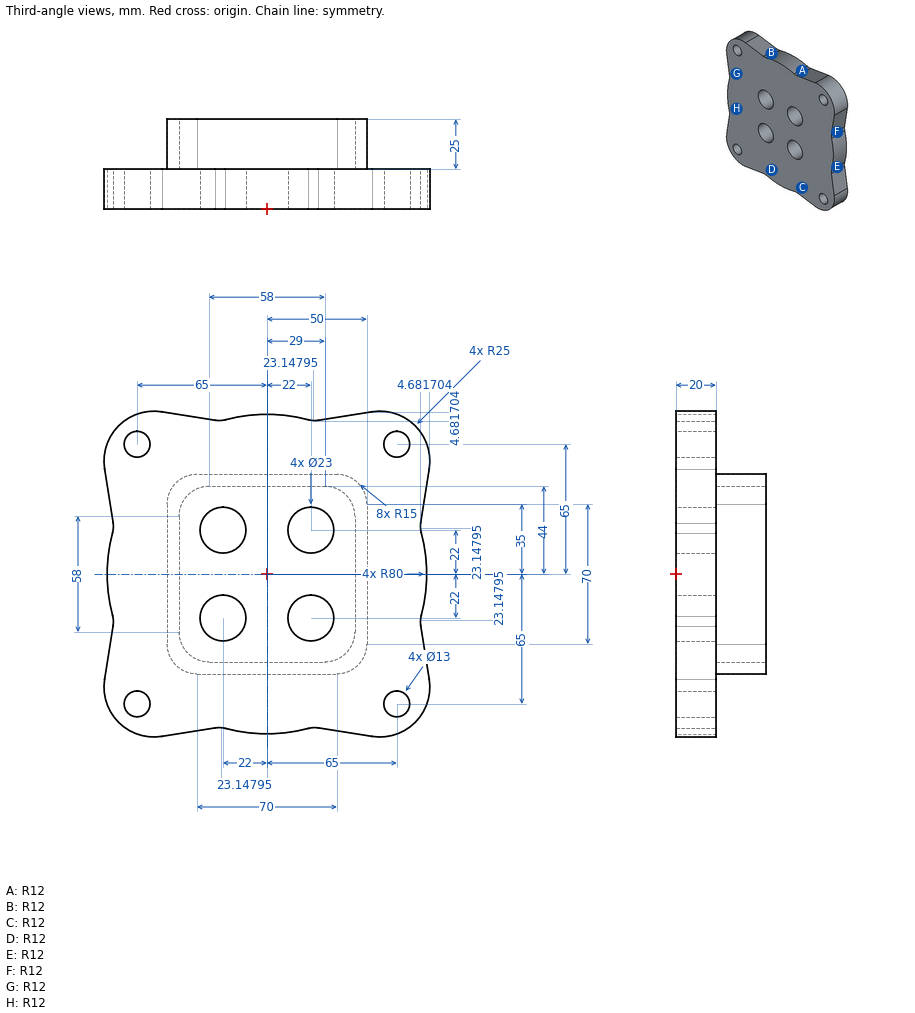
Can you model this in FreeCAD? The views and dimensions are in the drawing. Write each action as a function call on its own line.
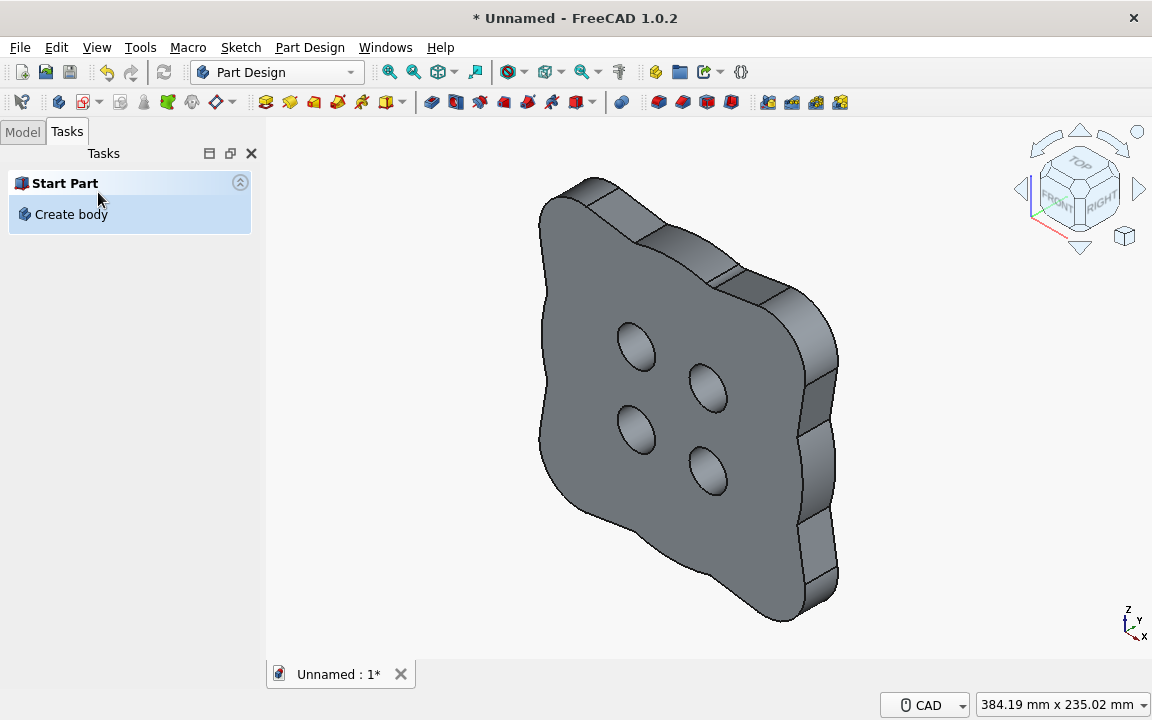
key(2)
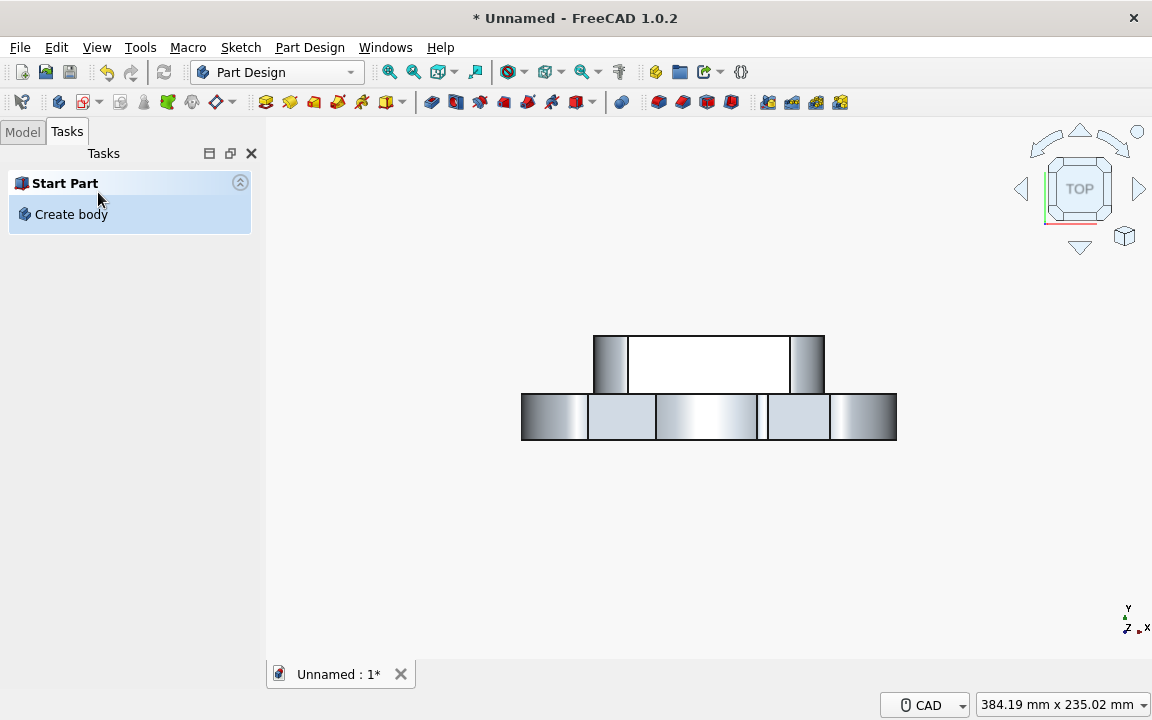
click(390, 72)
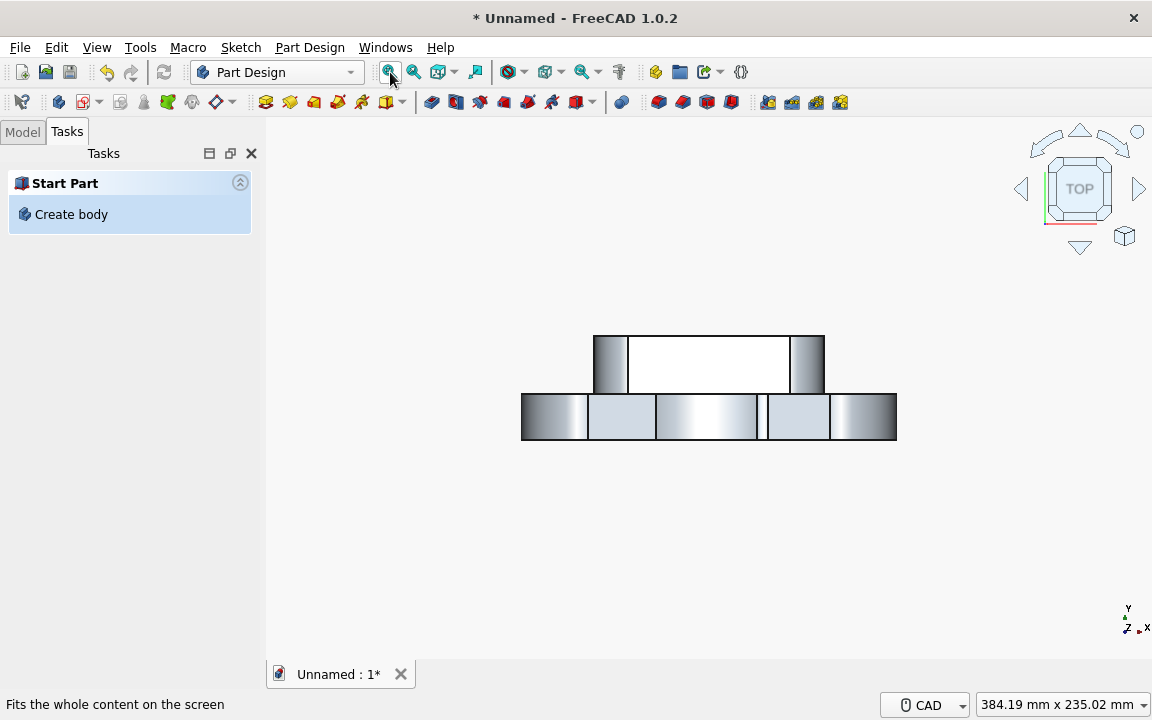
key(0)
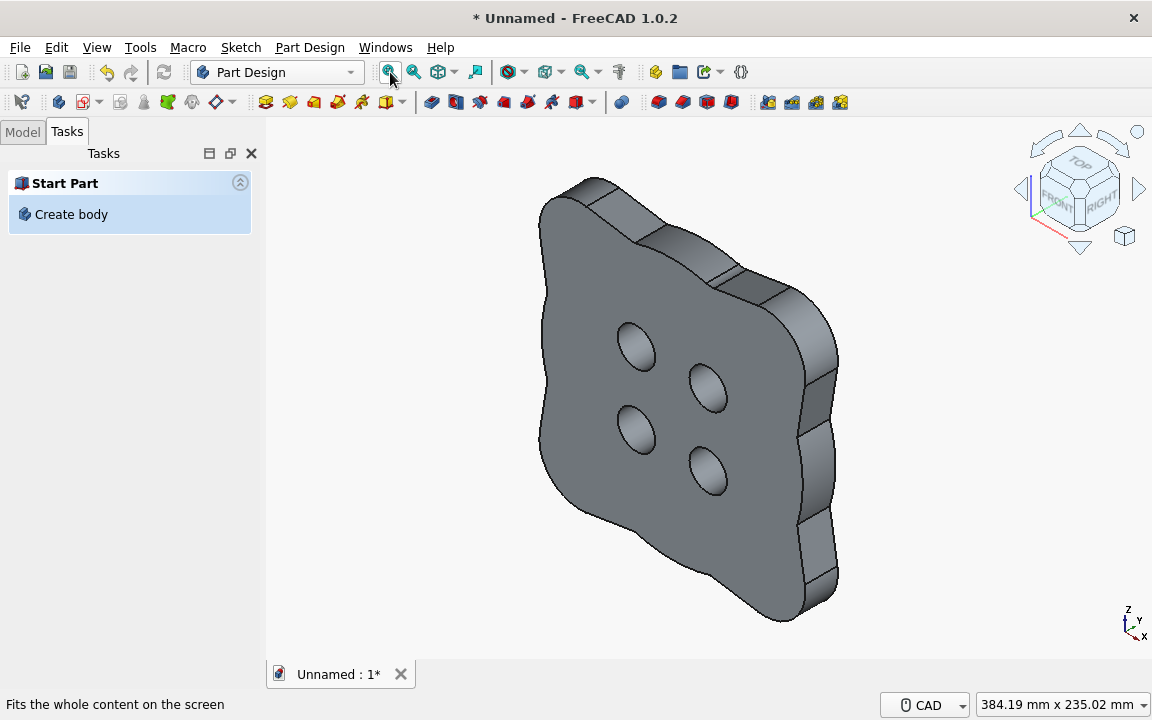
key(1)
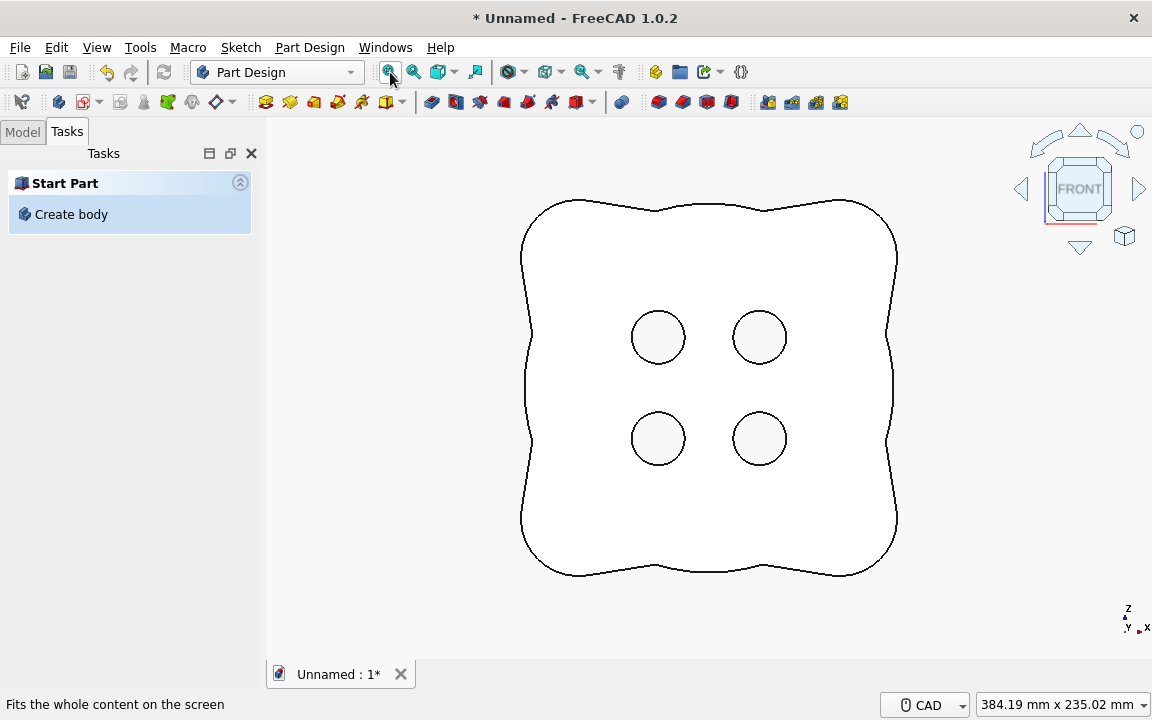
key(3)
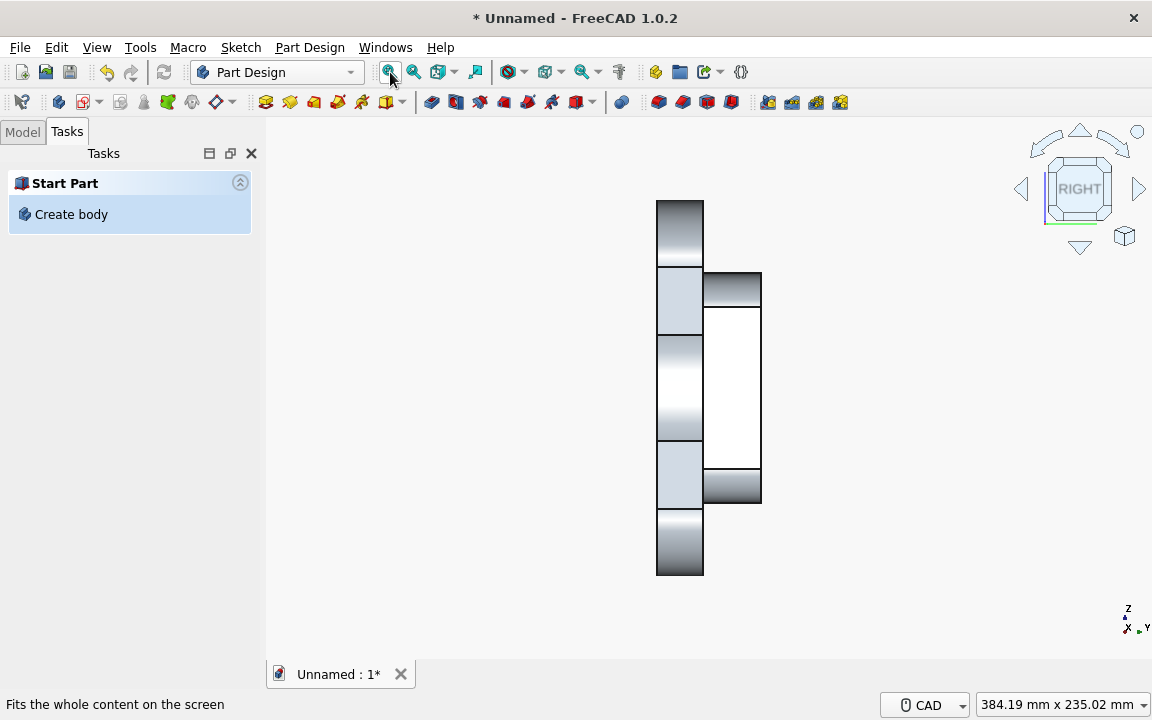
key(5)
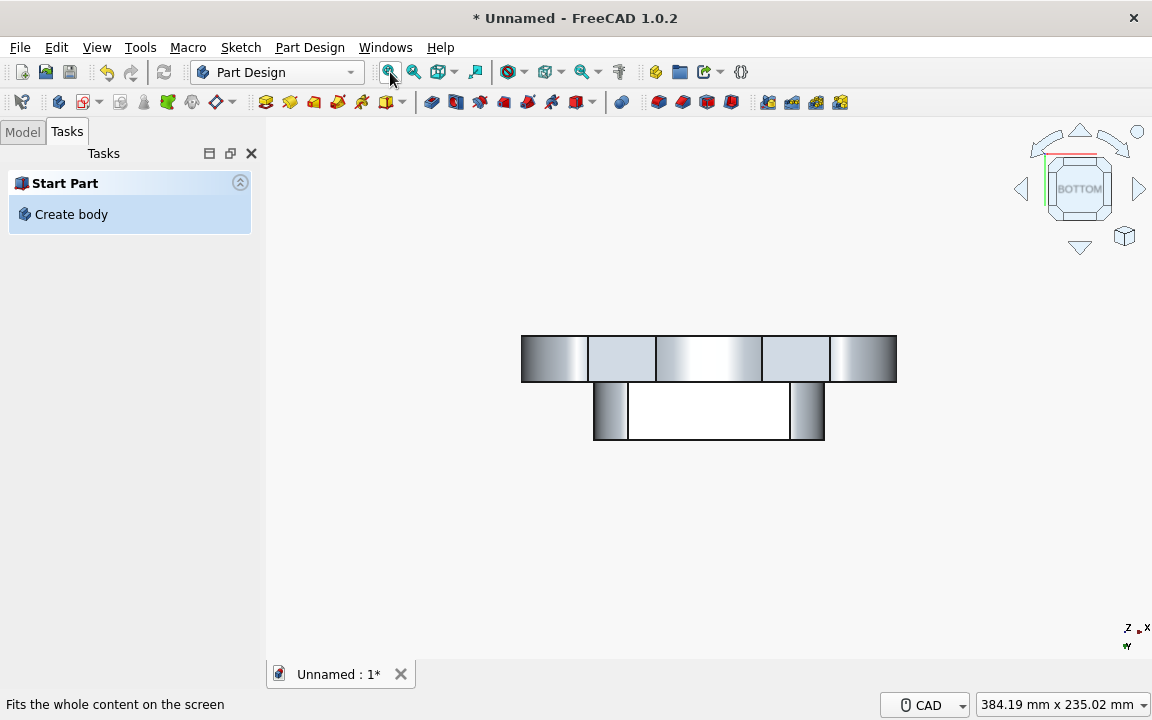
click(390, 72)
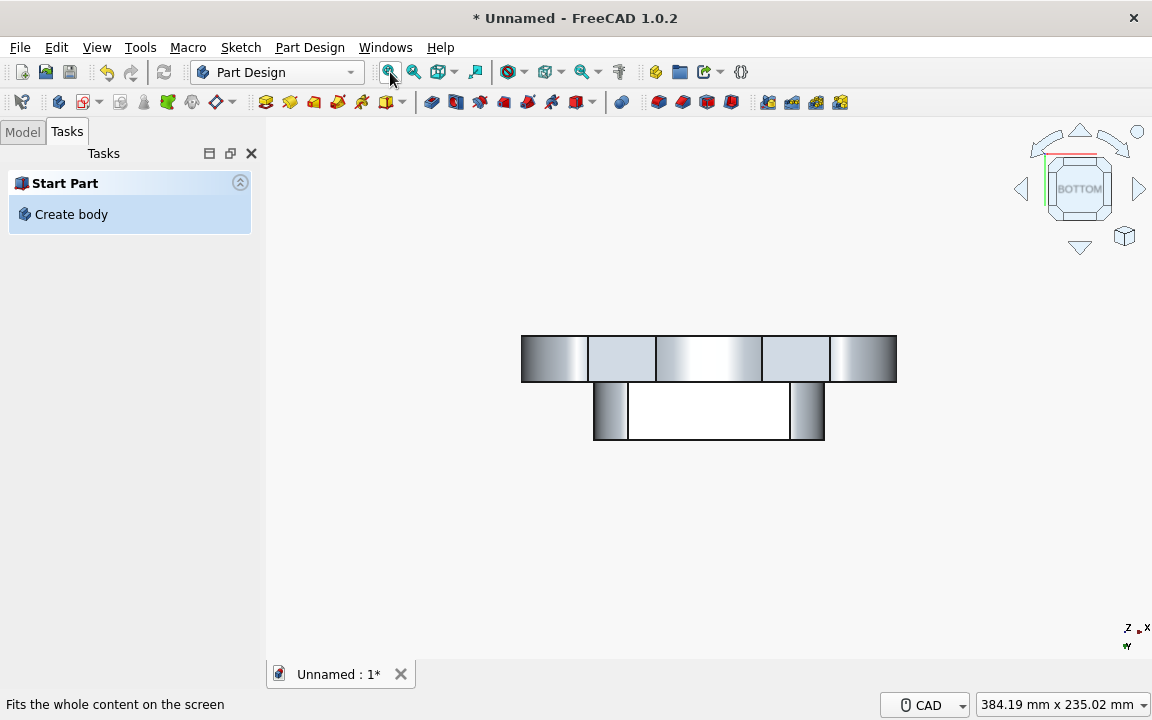
key(4)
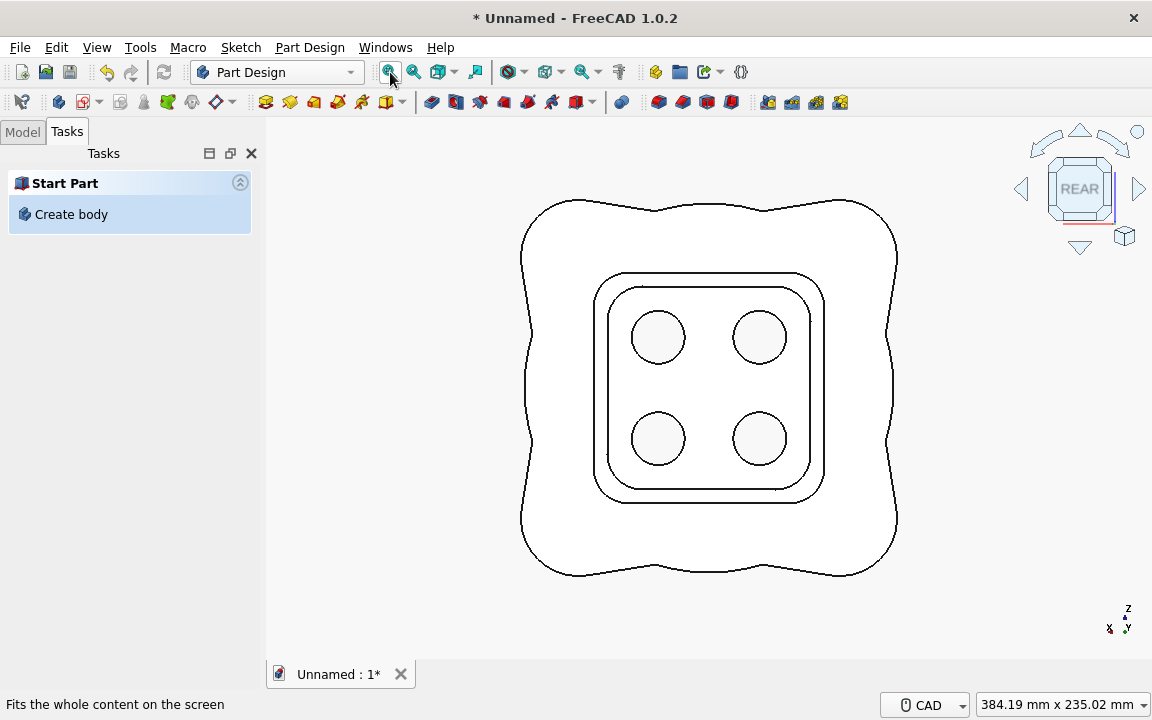
key(6)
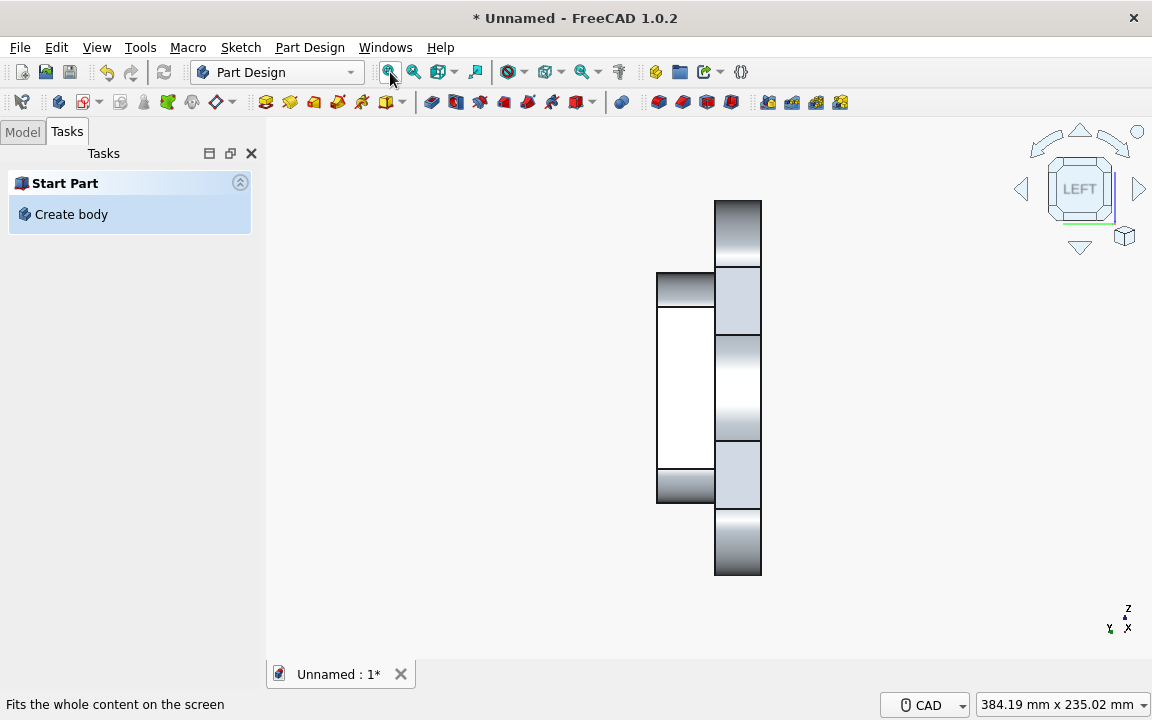
key(v)
key(3)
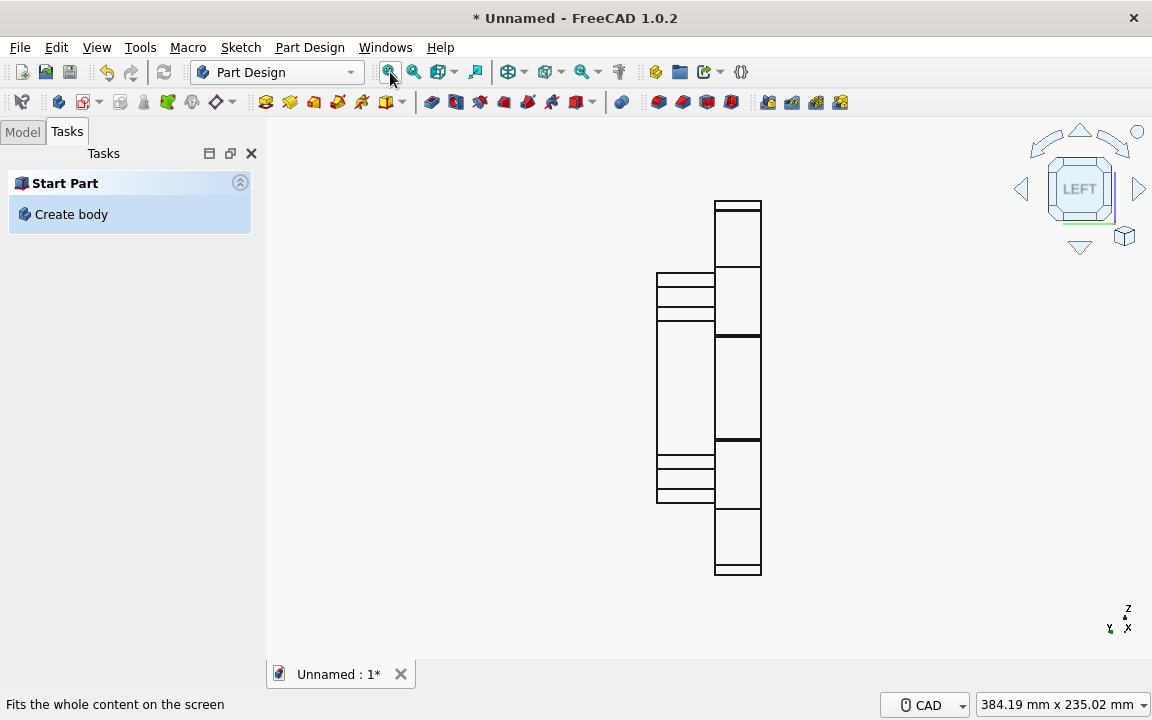
key(0)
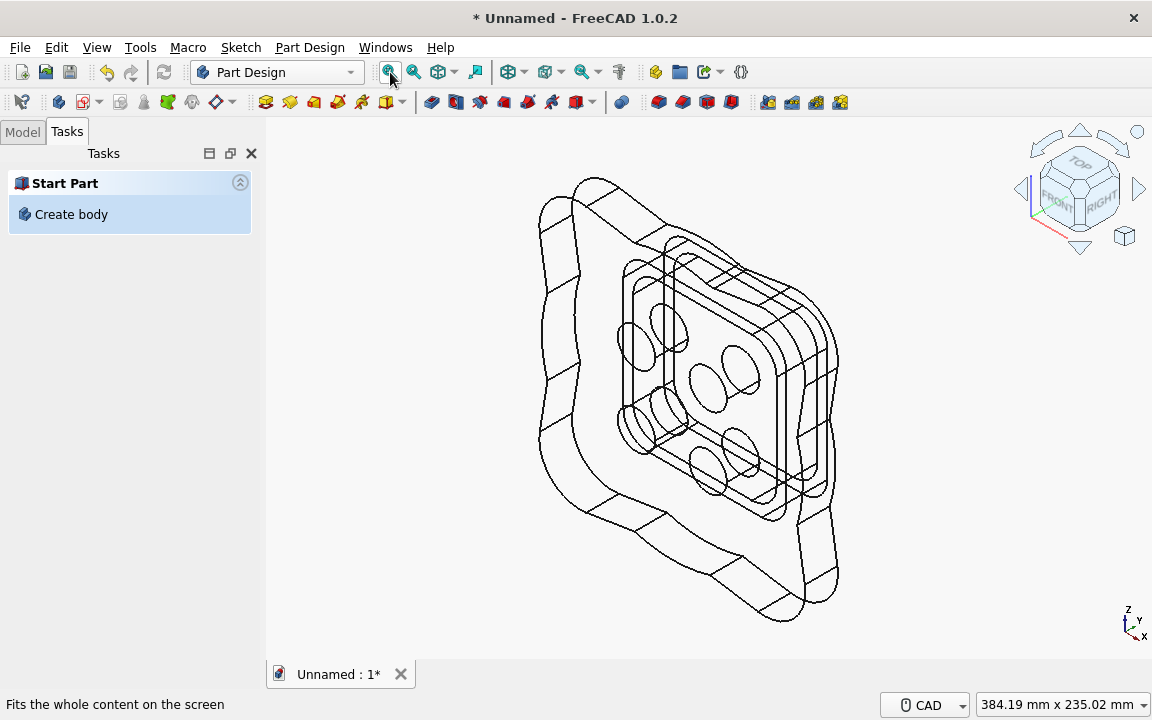
click(651, 233)